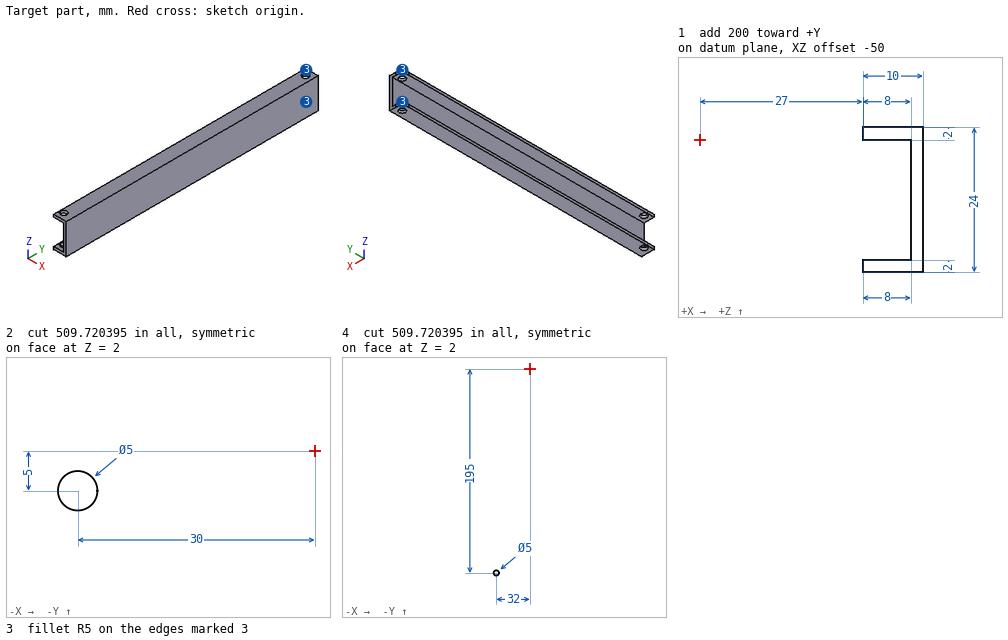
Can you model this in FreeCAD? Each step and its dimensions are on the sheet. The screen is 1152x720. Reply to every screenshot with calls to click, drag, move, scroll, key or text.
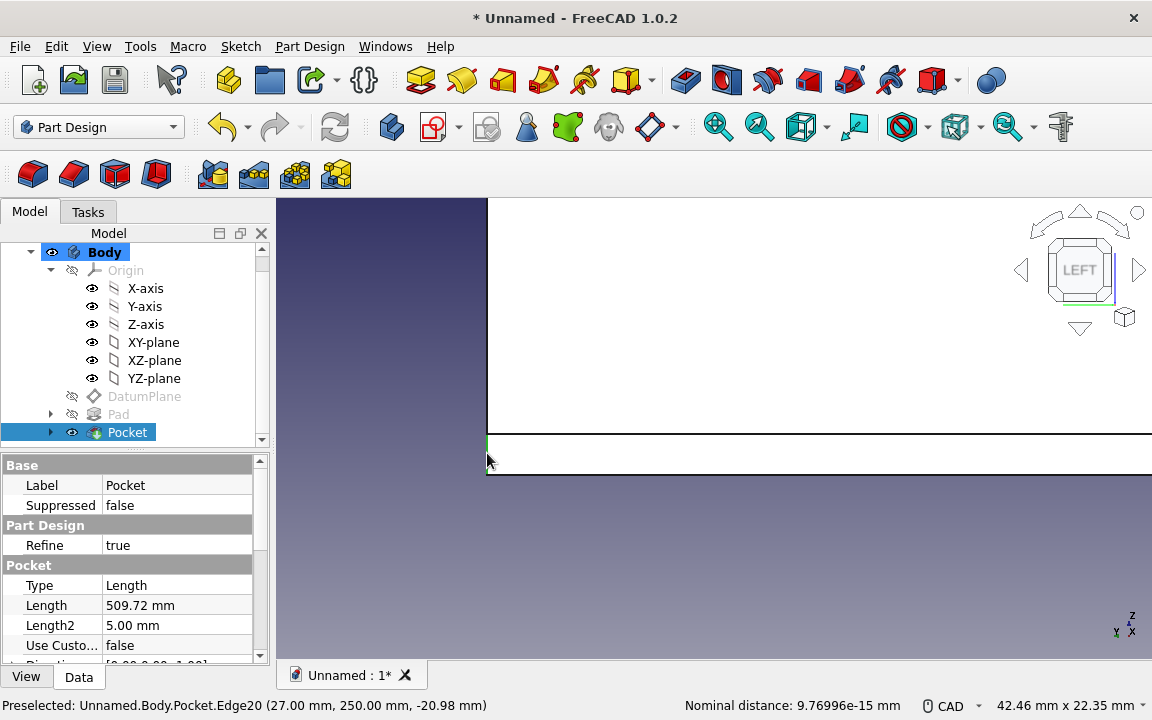
click(33, 174)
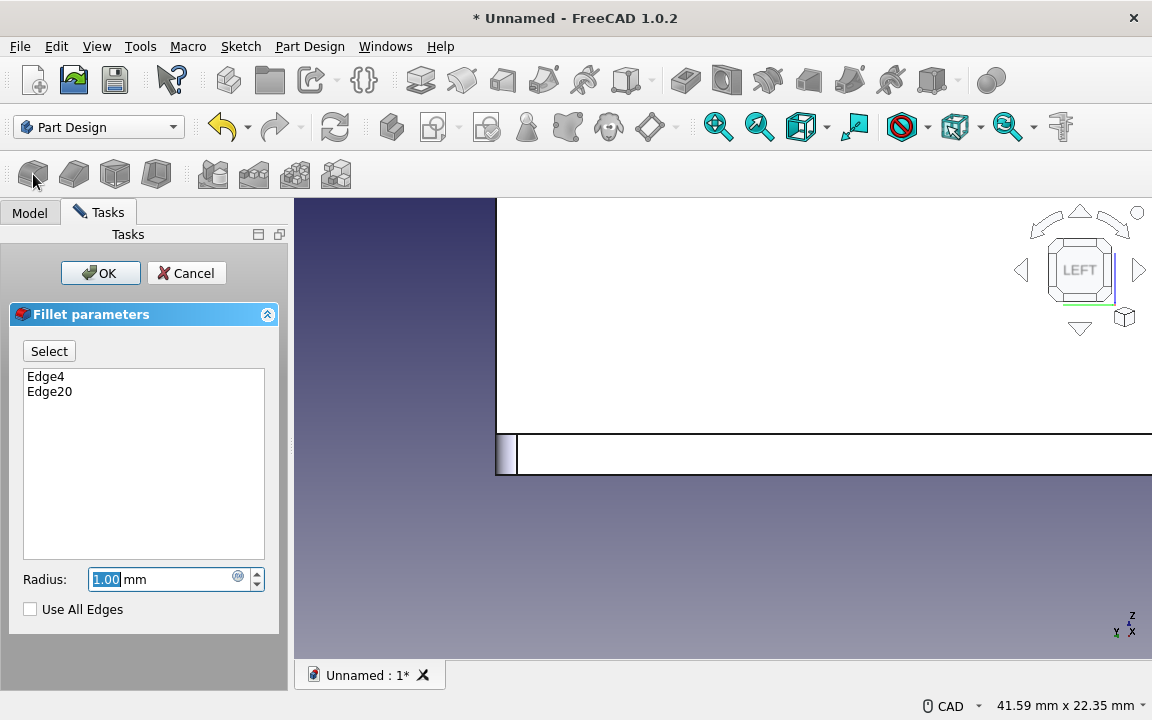
text(5)
key(Tab)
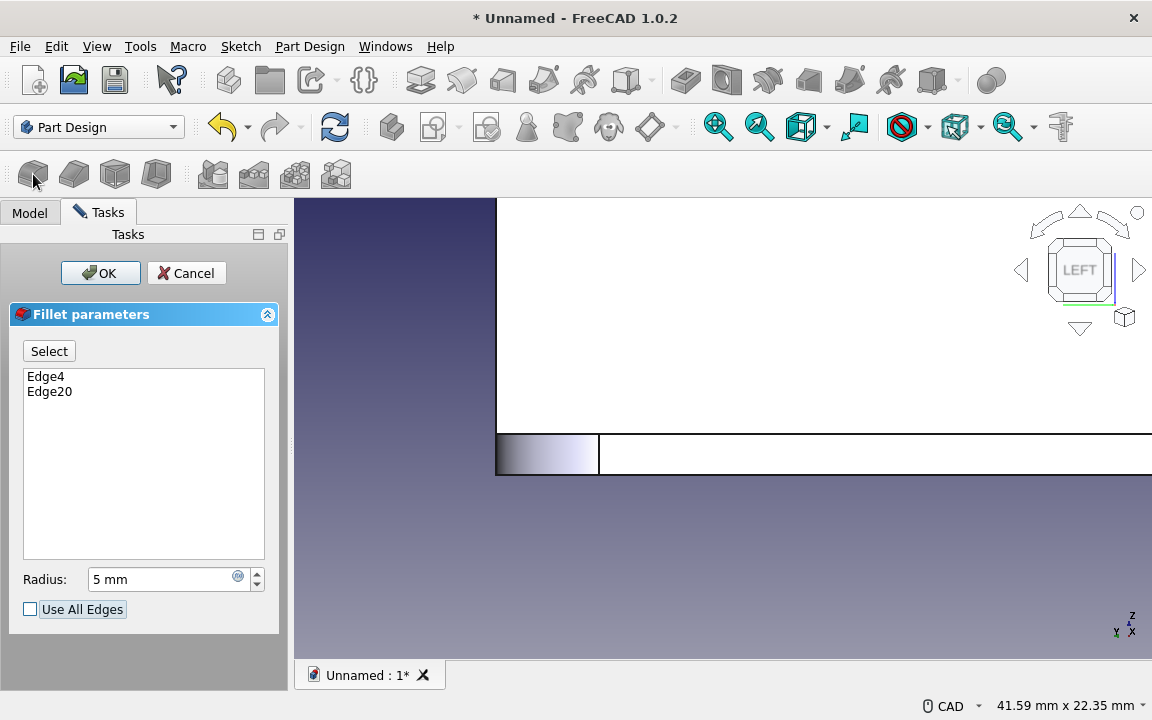
click(101, 273)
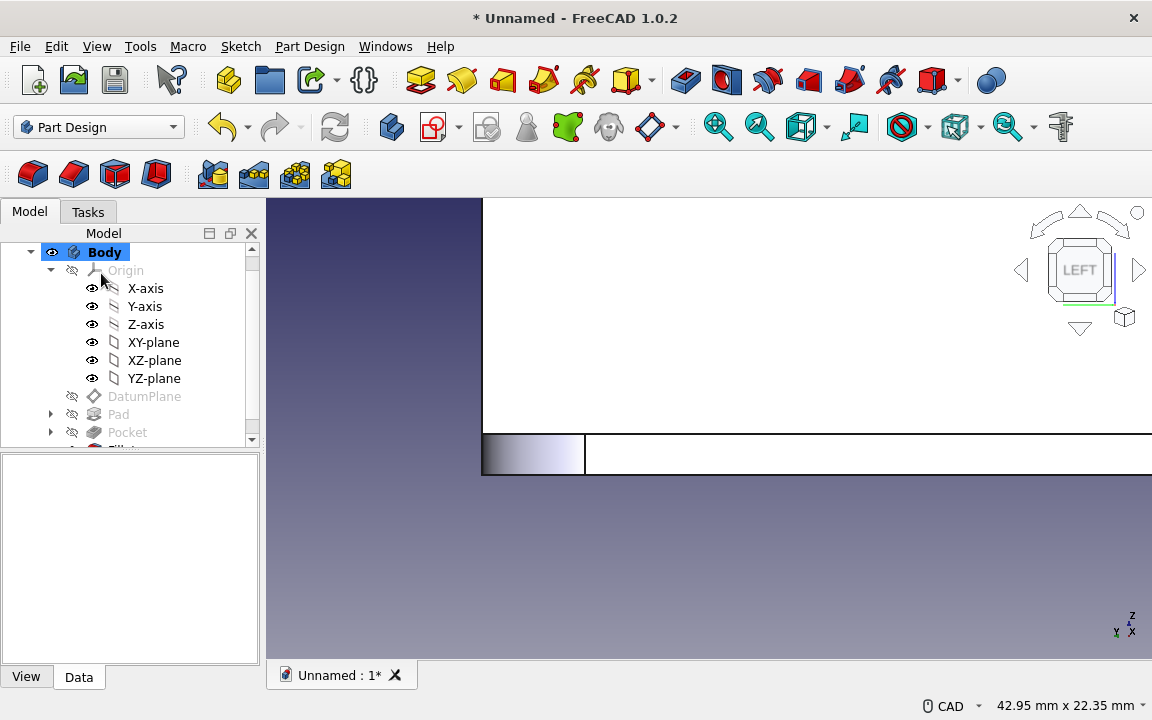
click(719, 128)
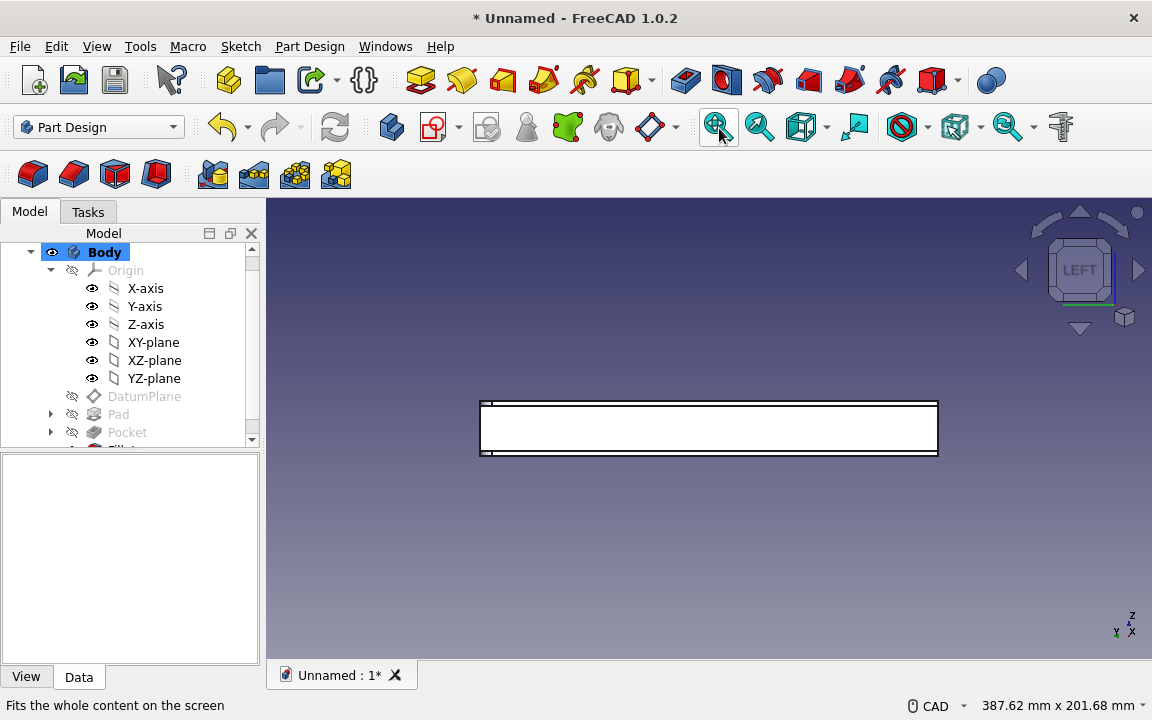
key(0)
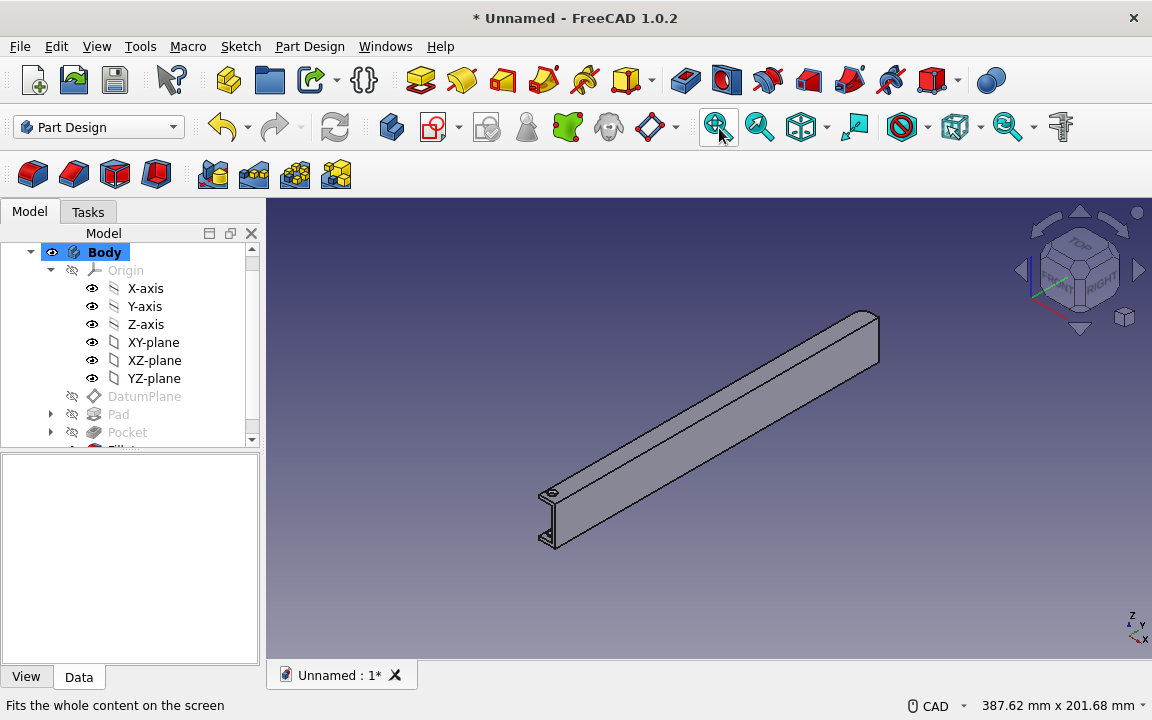
click(845, 324)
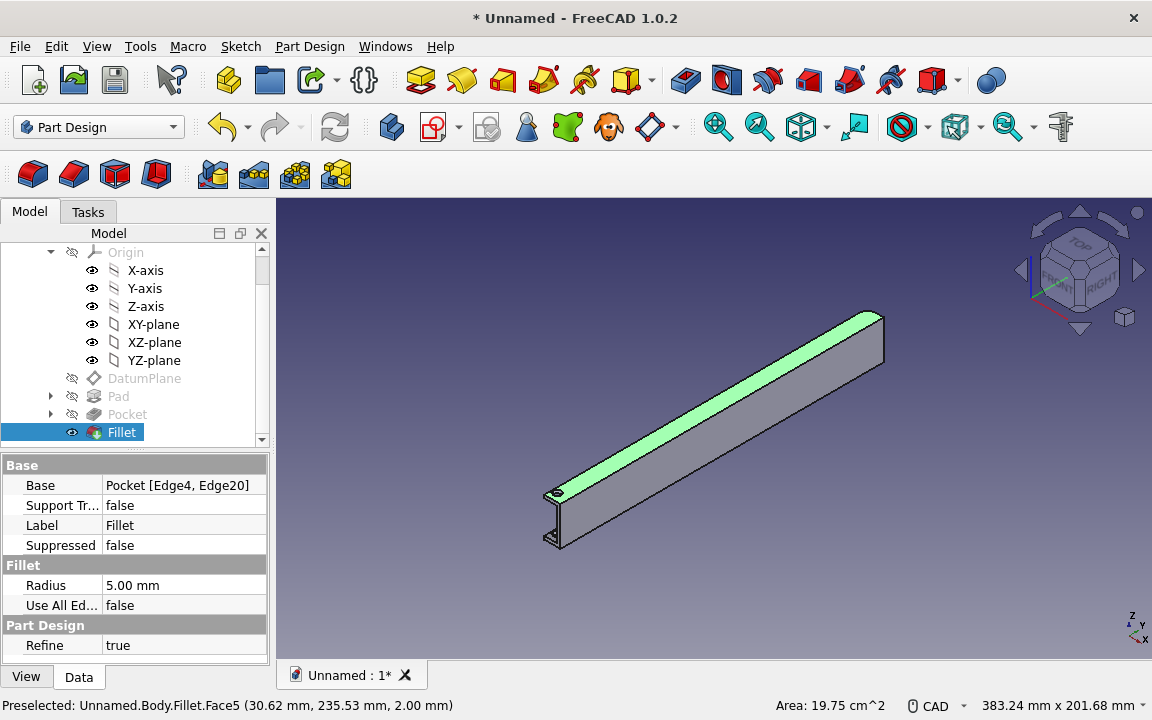
click(432, 128)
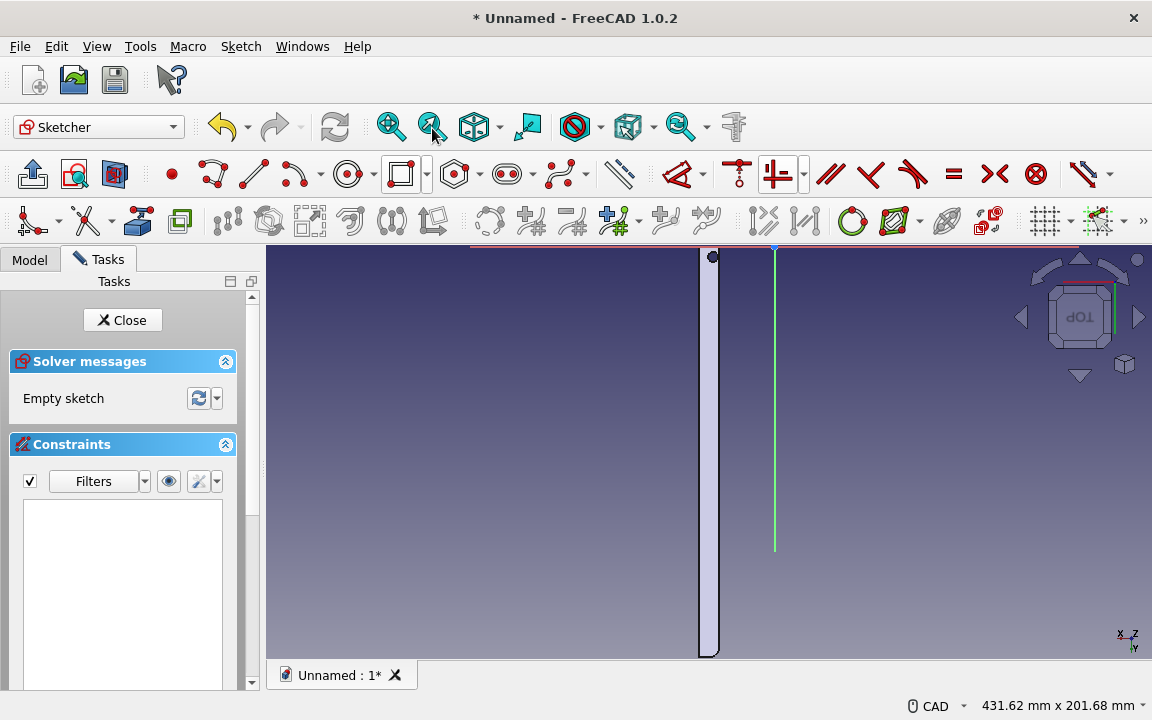
scroll(640, 452, down, 5)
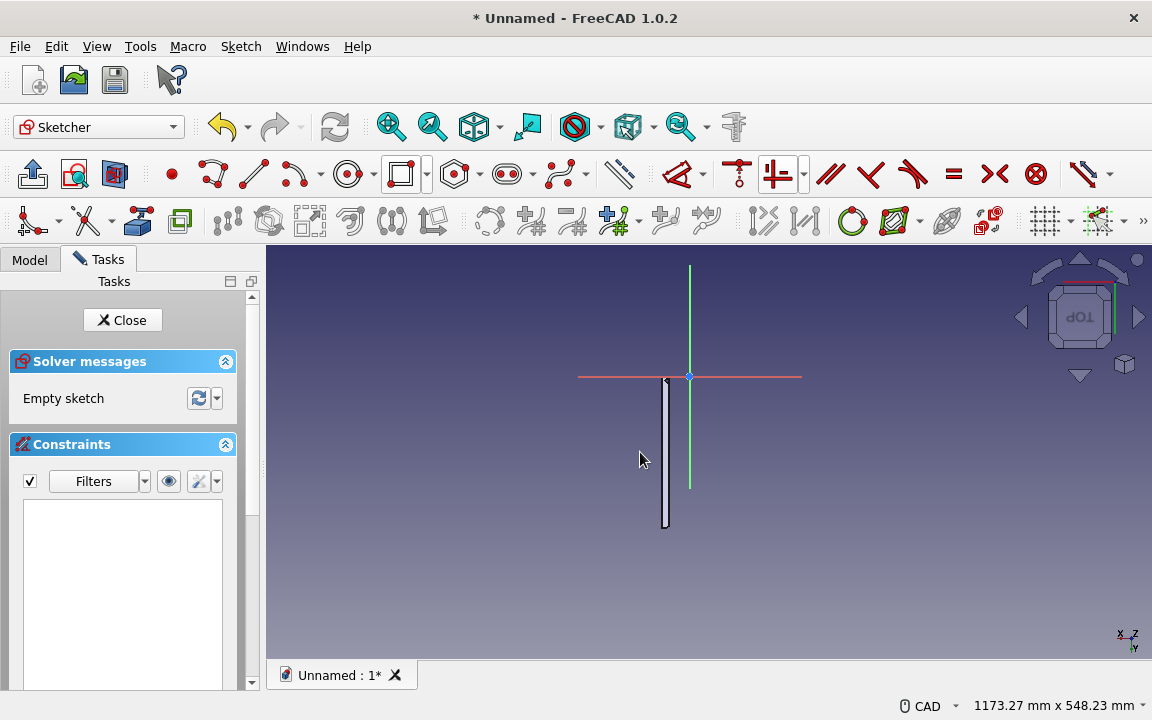
scroll(667, 528, up, 15)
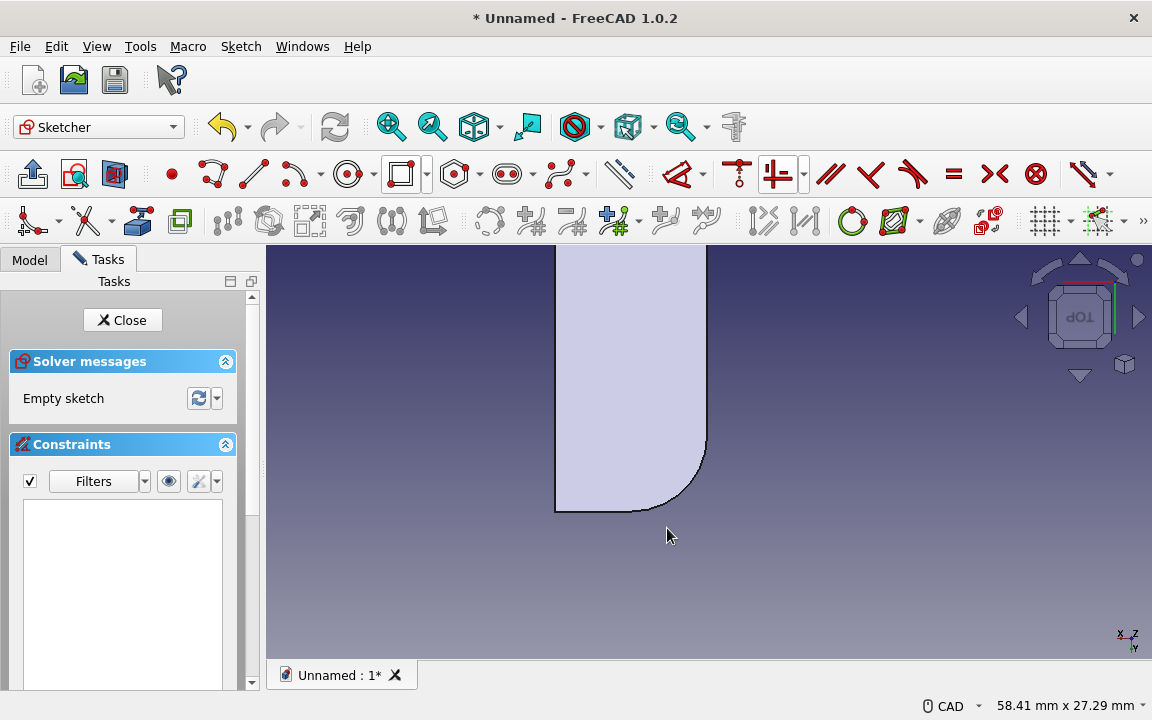
scroll(627, 429, up, 6)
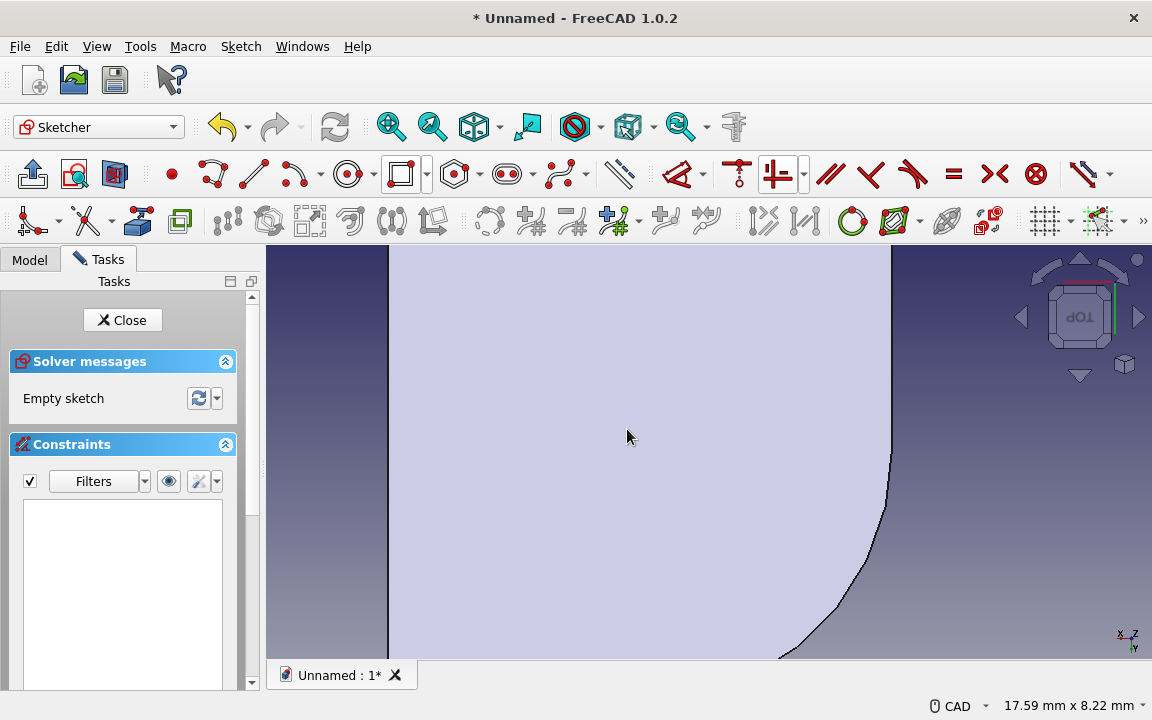
click(348, 174)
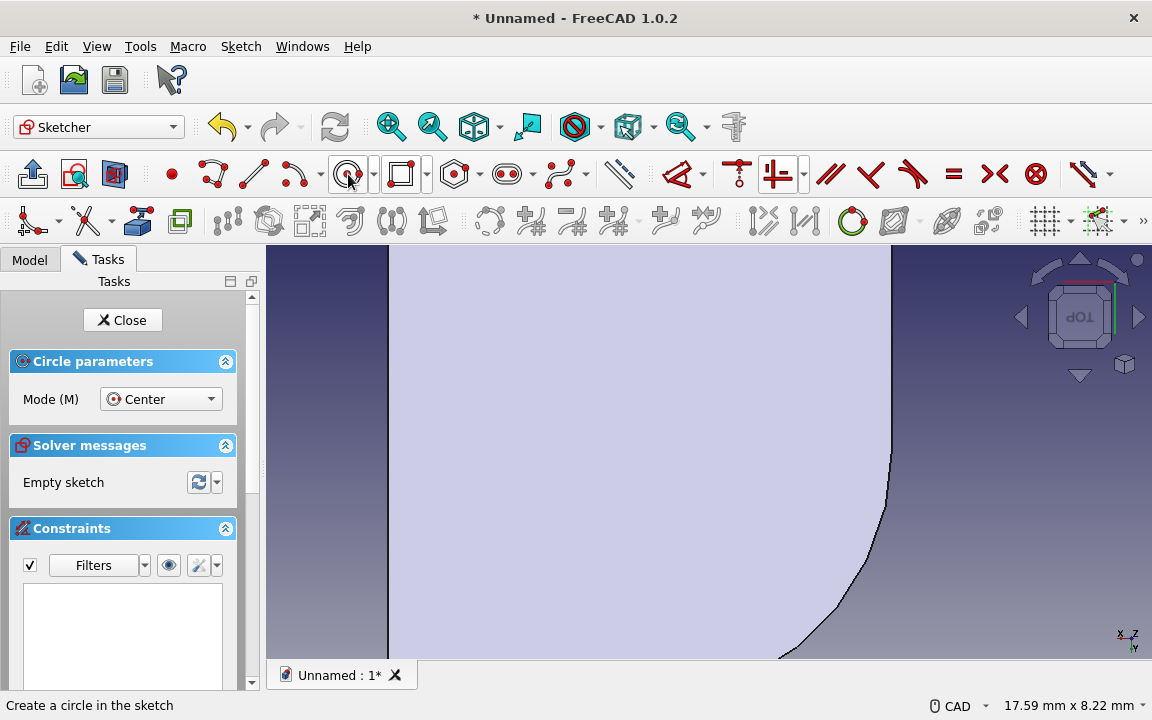
click(640, 450)
move(729, 361)